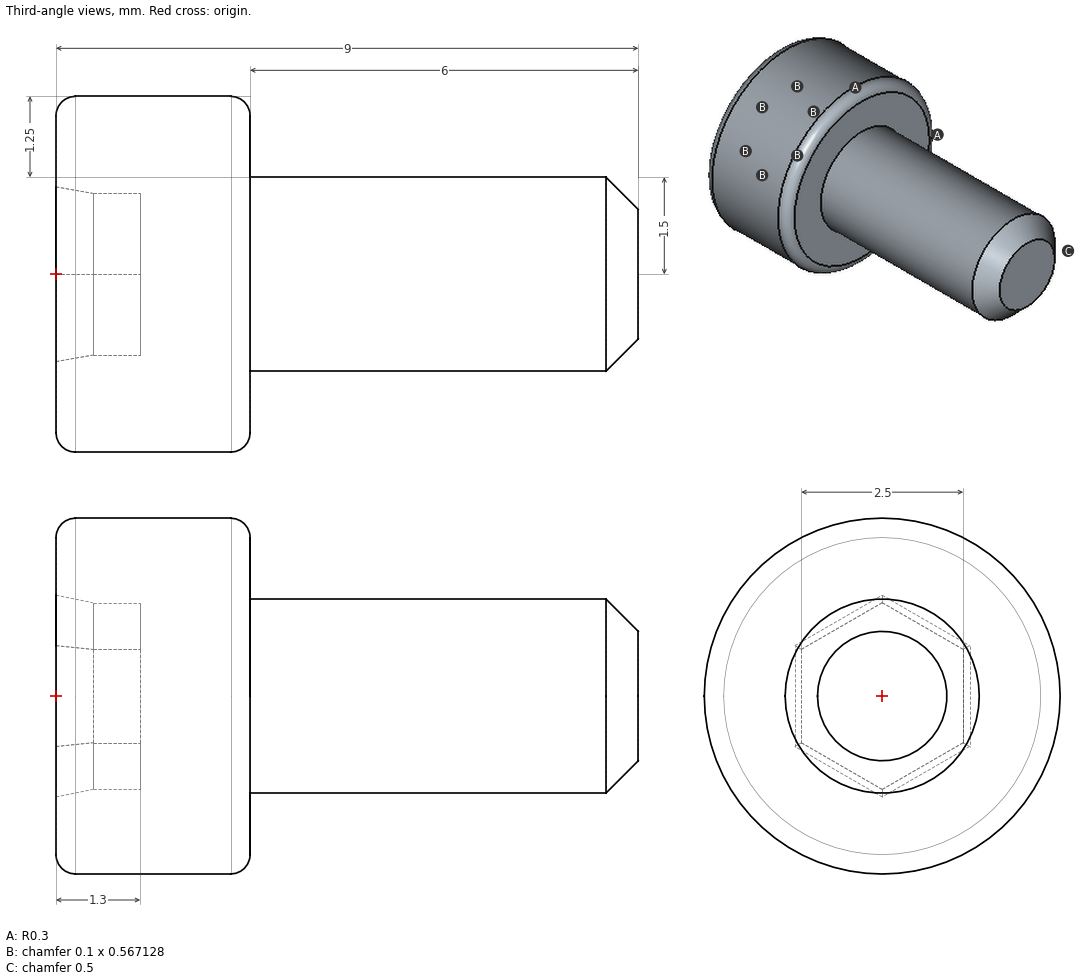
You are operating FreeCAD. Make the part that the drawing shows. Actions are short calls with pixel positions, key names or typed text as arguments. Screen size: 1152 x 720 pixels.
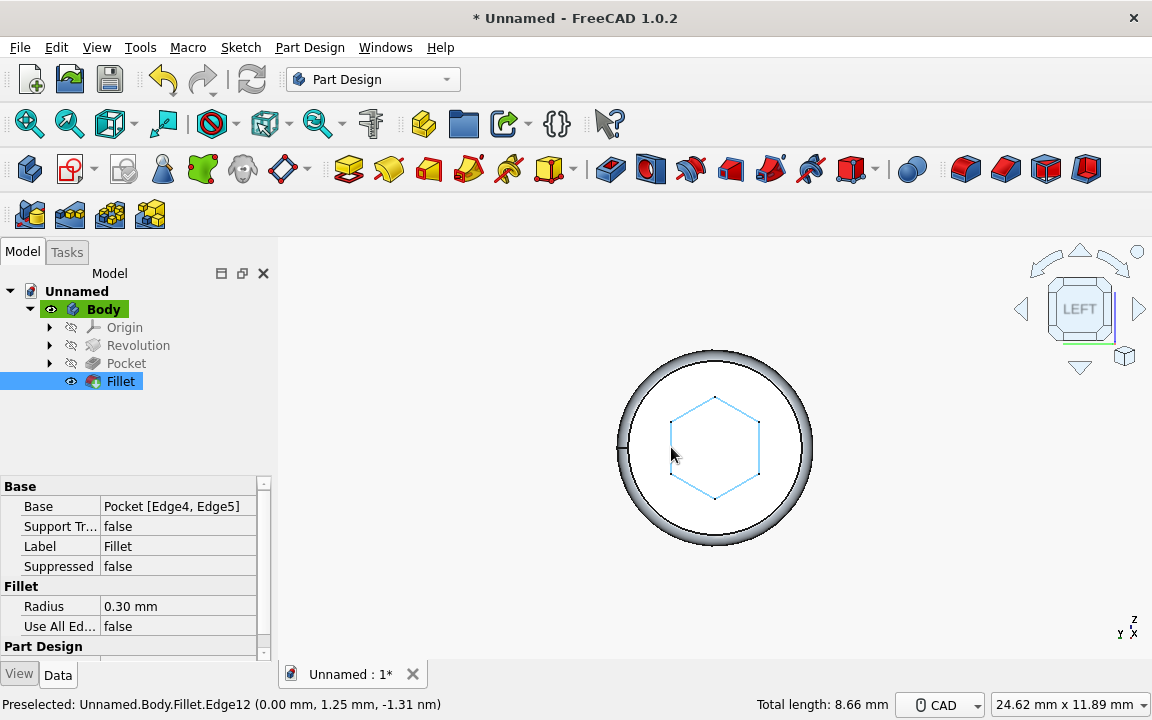
click(1006, 170)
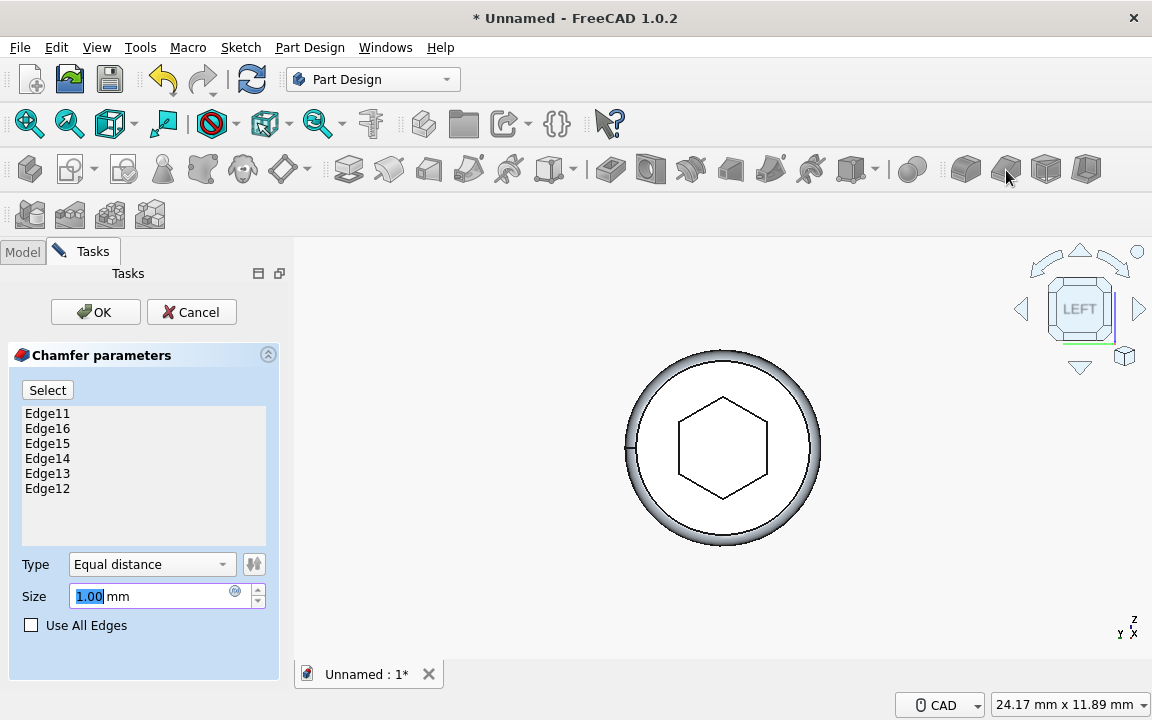
text(0.1)
key(Tab)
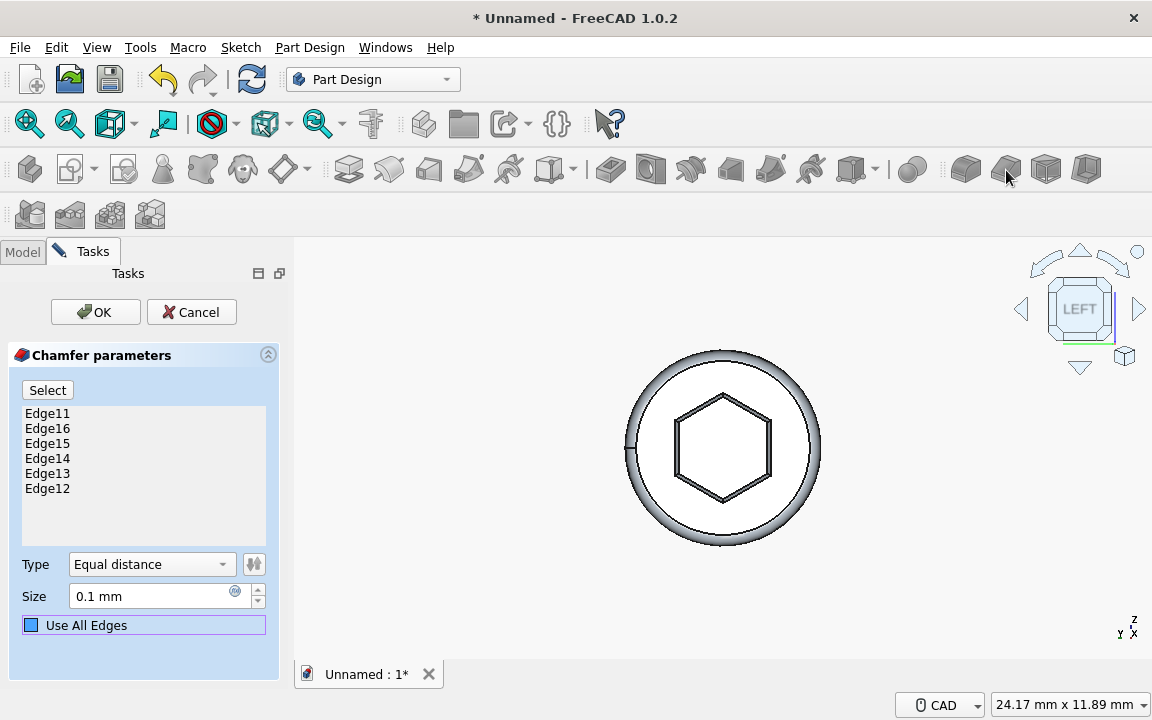
click(153, 564)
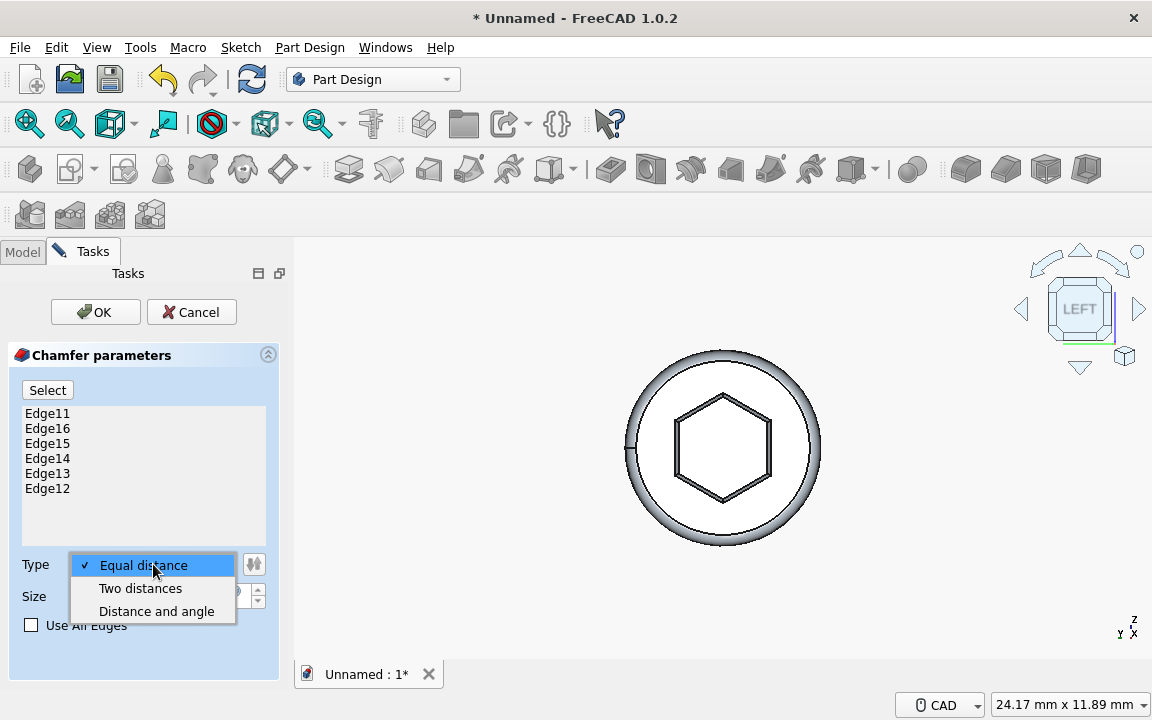
click(152, 588)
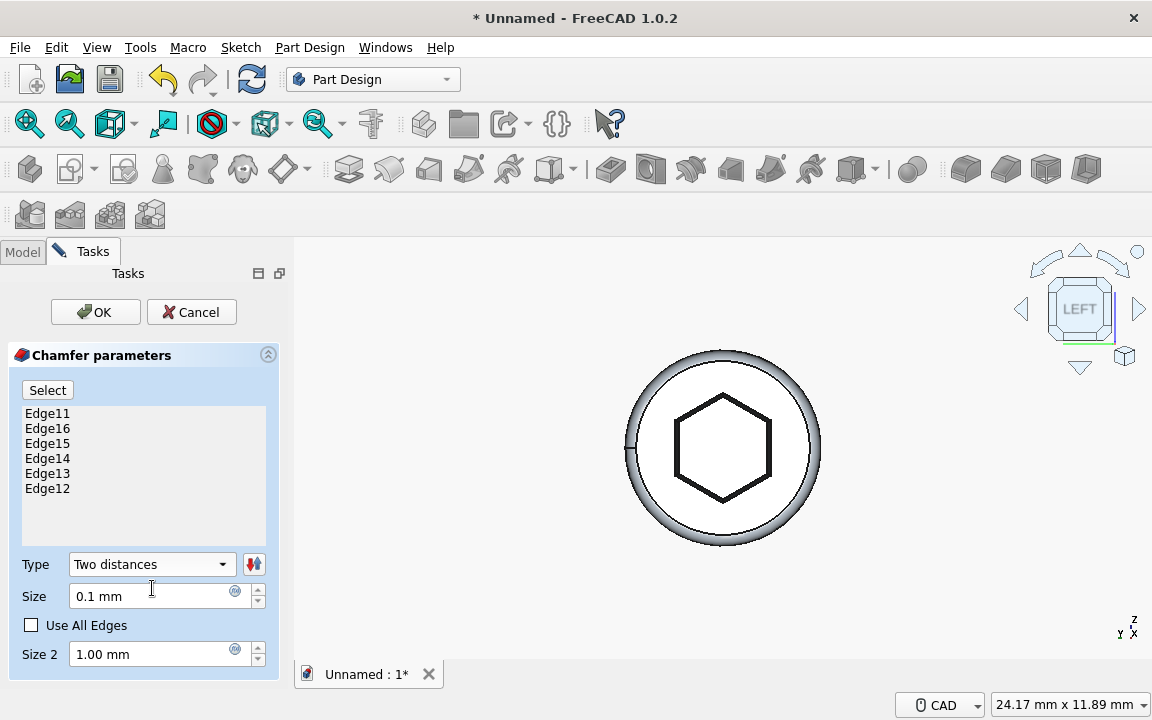
triple_click(160, 654)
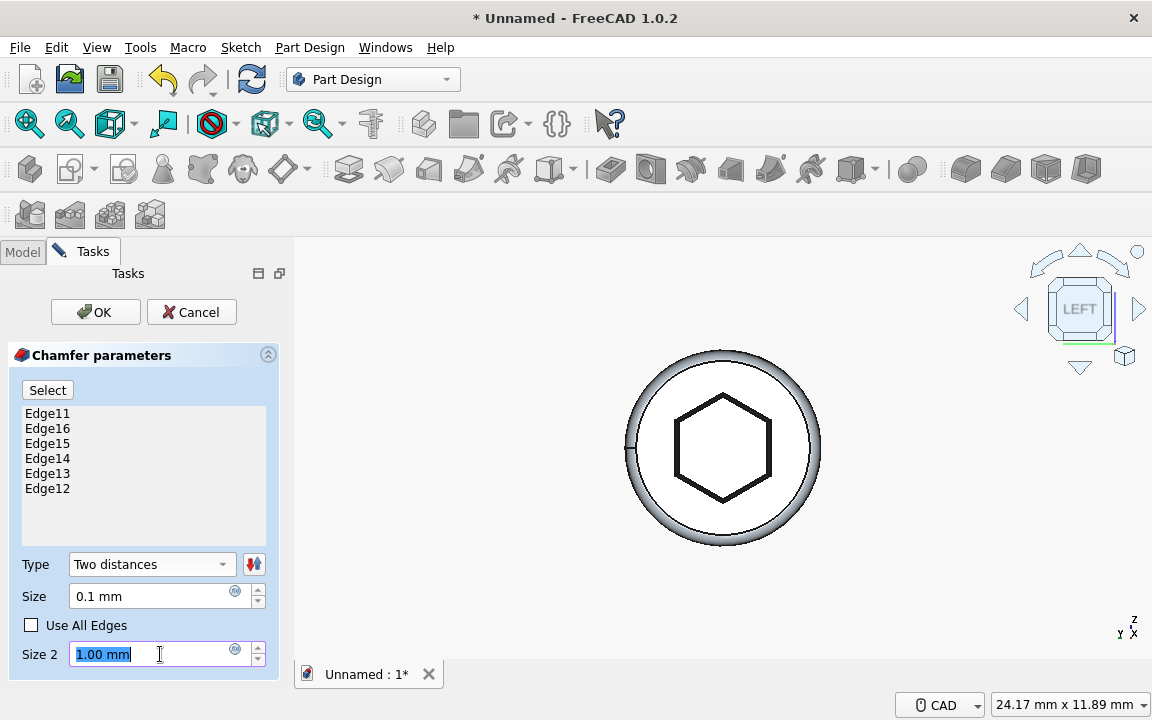
text(0.567128)
key(Tab)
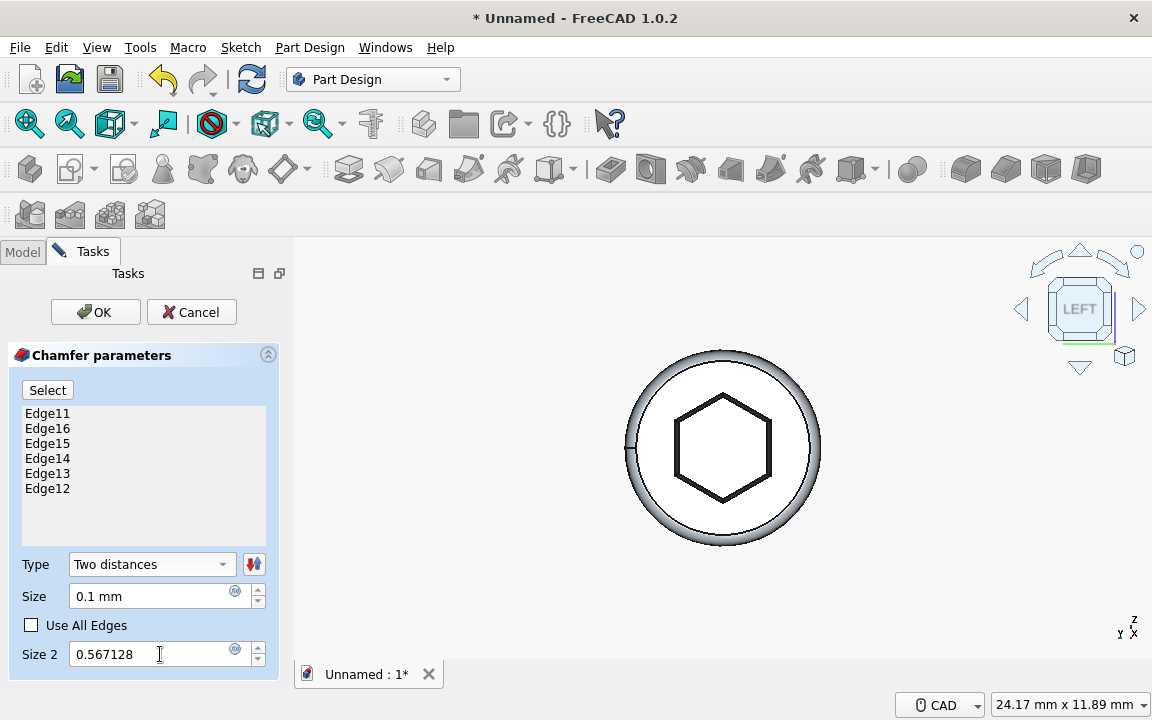
click(96, 312)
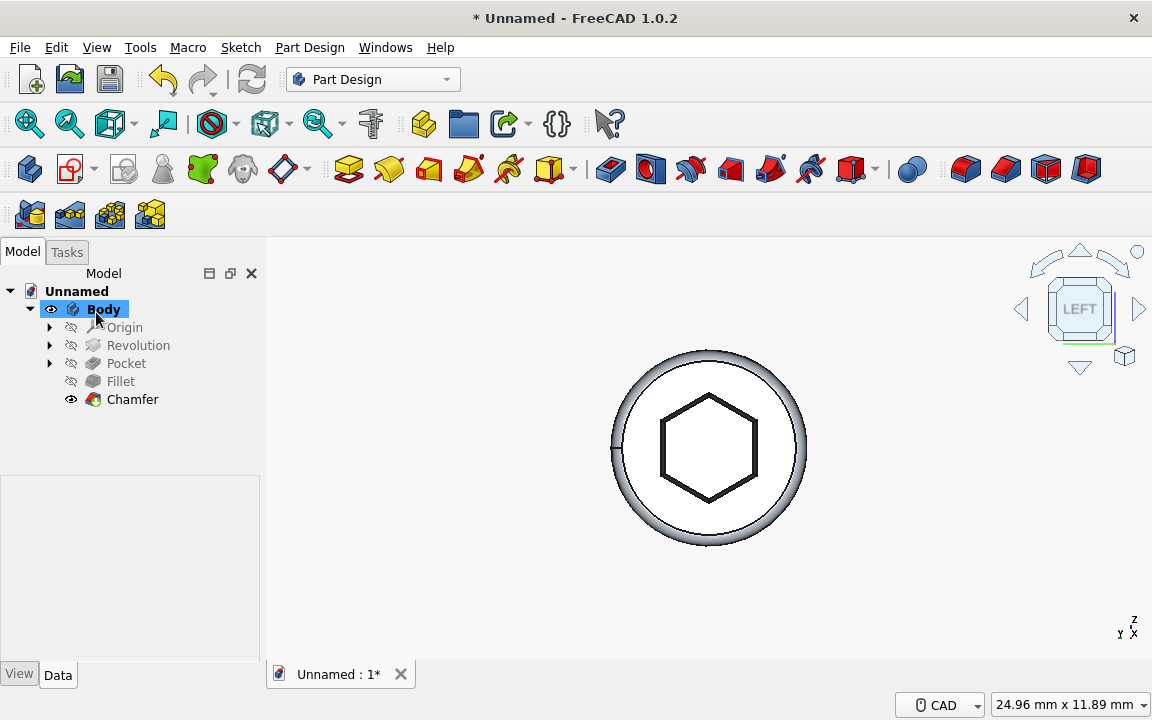
key(0)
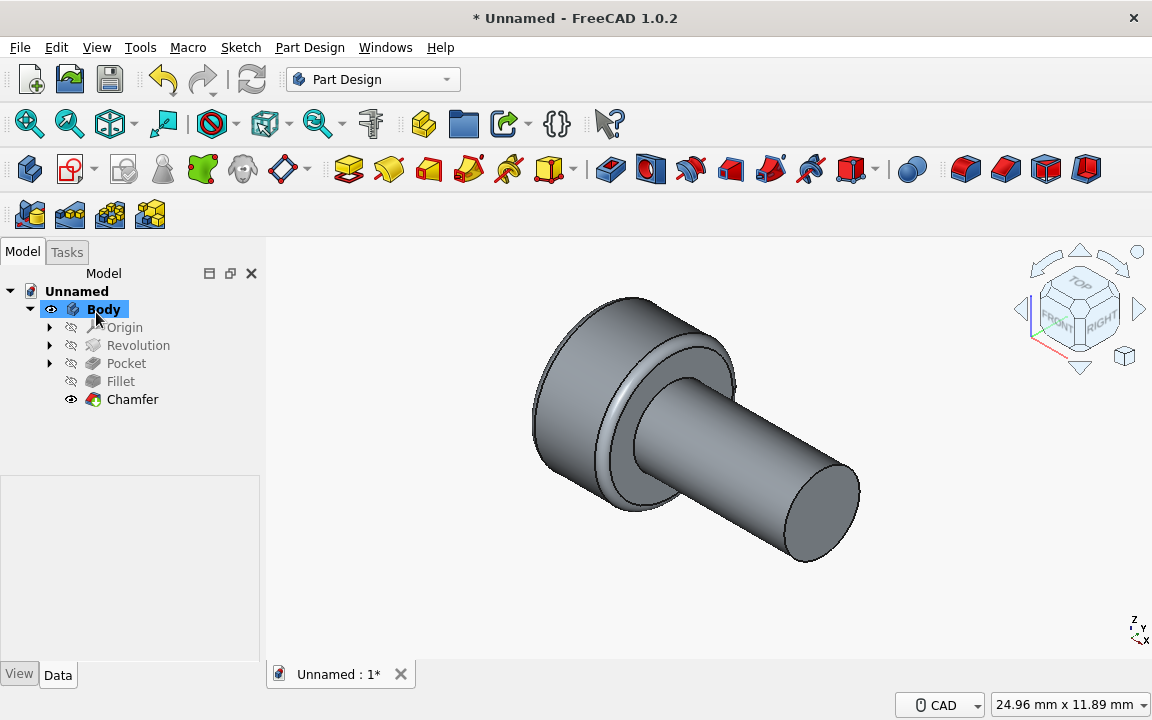
click(784, 534)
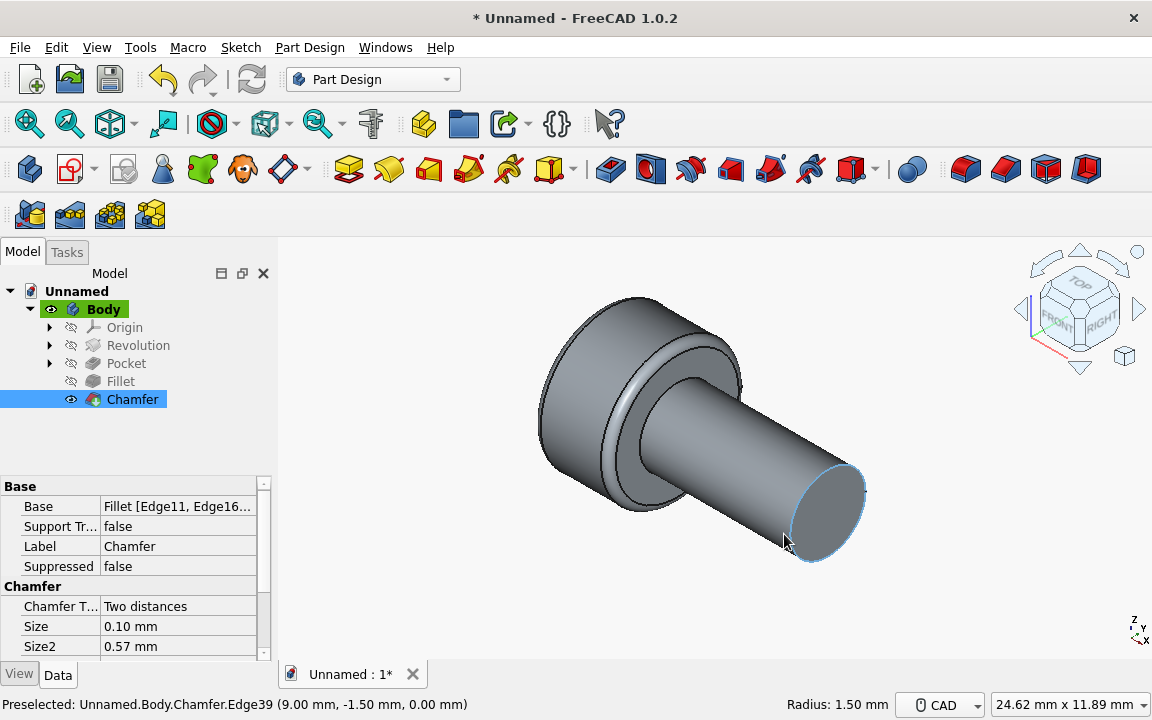
click(1006, 170)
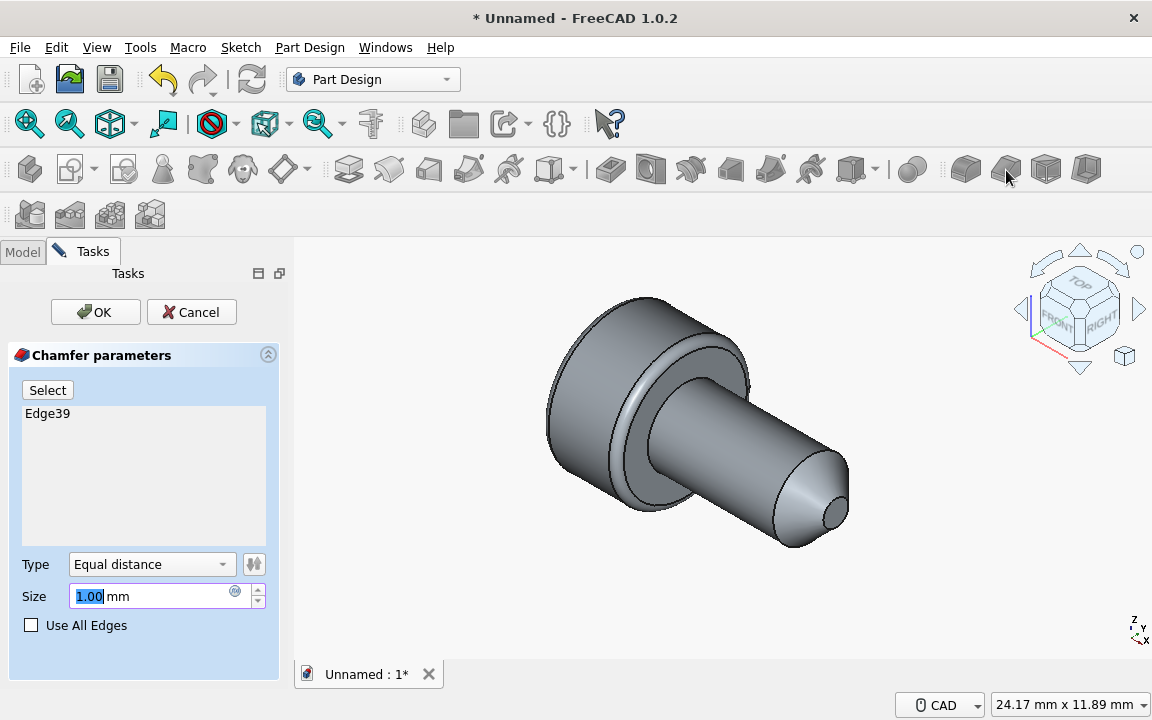
text(0.5)
key(Tab)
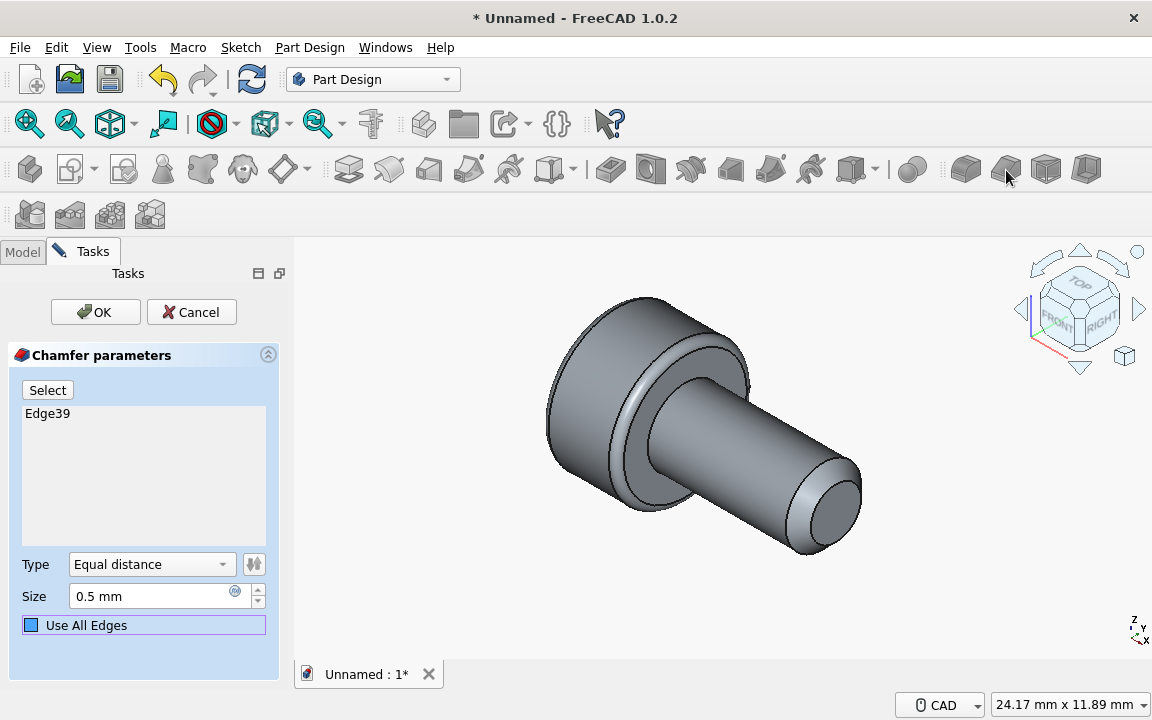
click(96, 312)